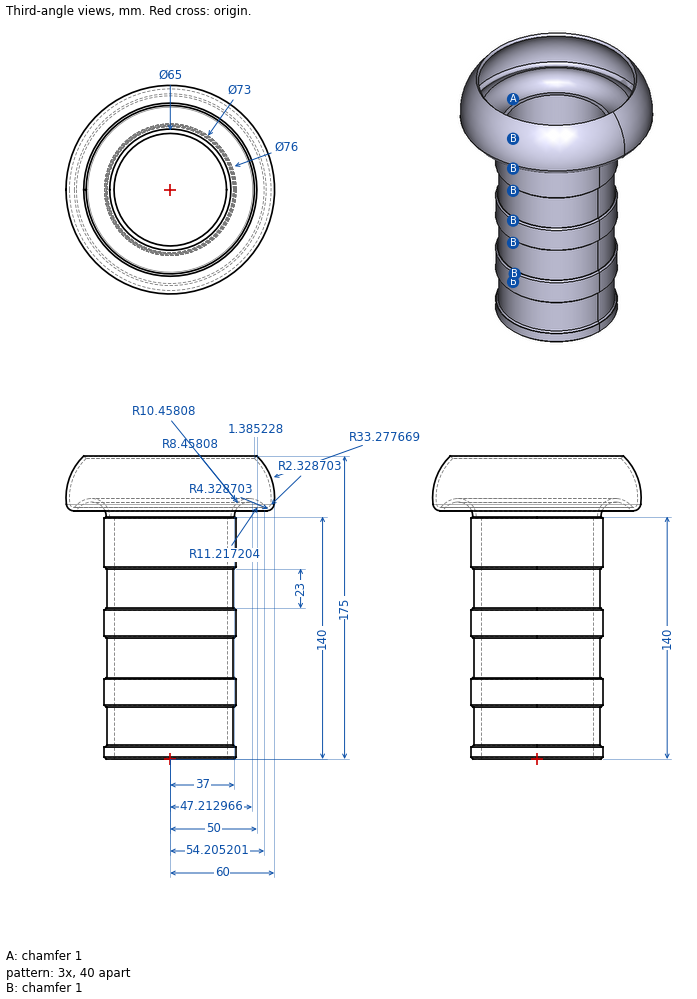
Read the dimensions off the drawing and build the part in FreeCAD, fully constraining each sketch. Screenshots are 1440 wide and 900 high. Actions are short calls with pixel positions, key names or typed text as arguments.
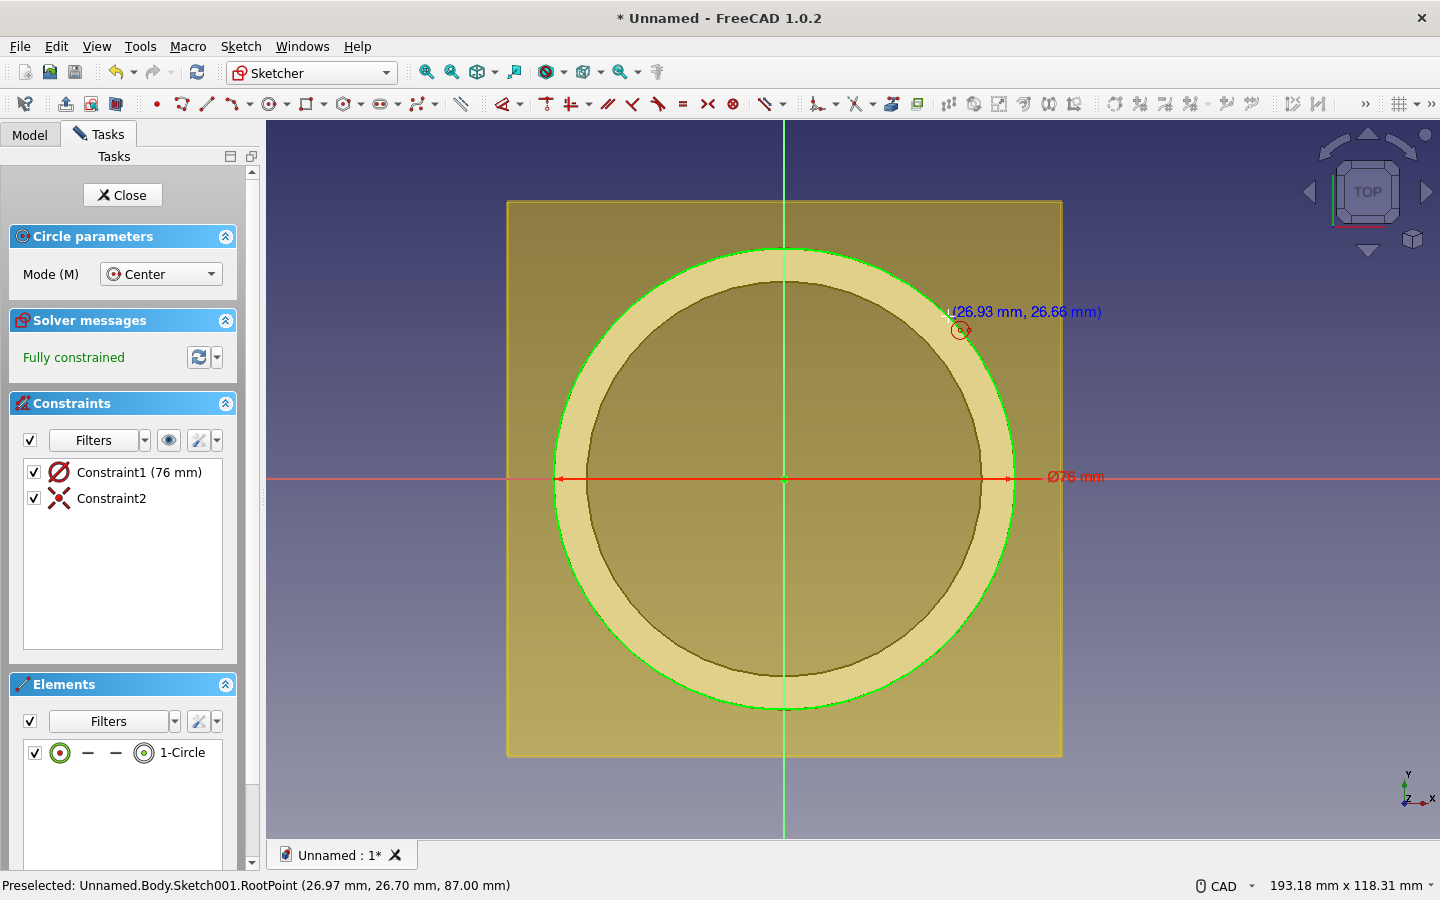
click(784, 479)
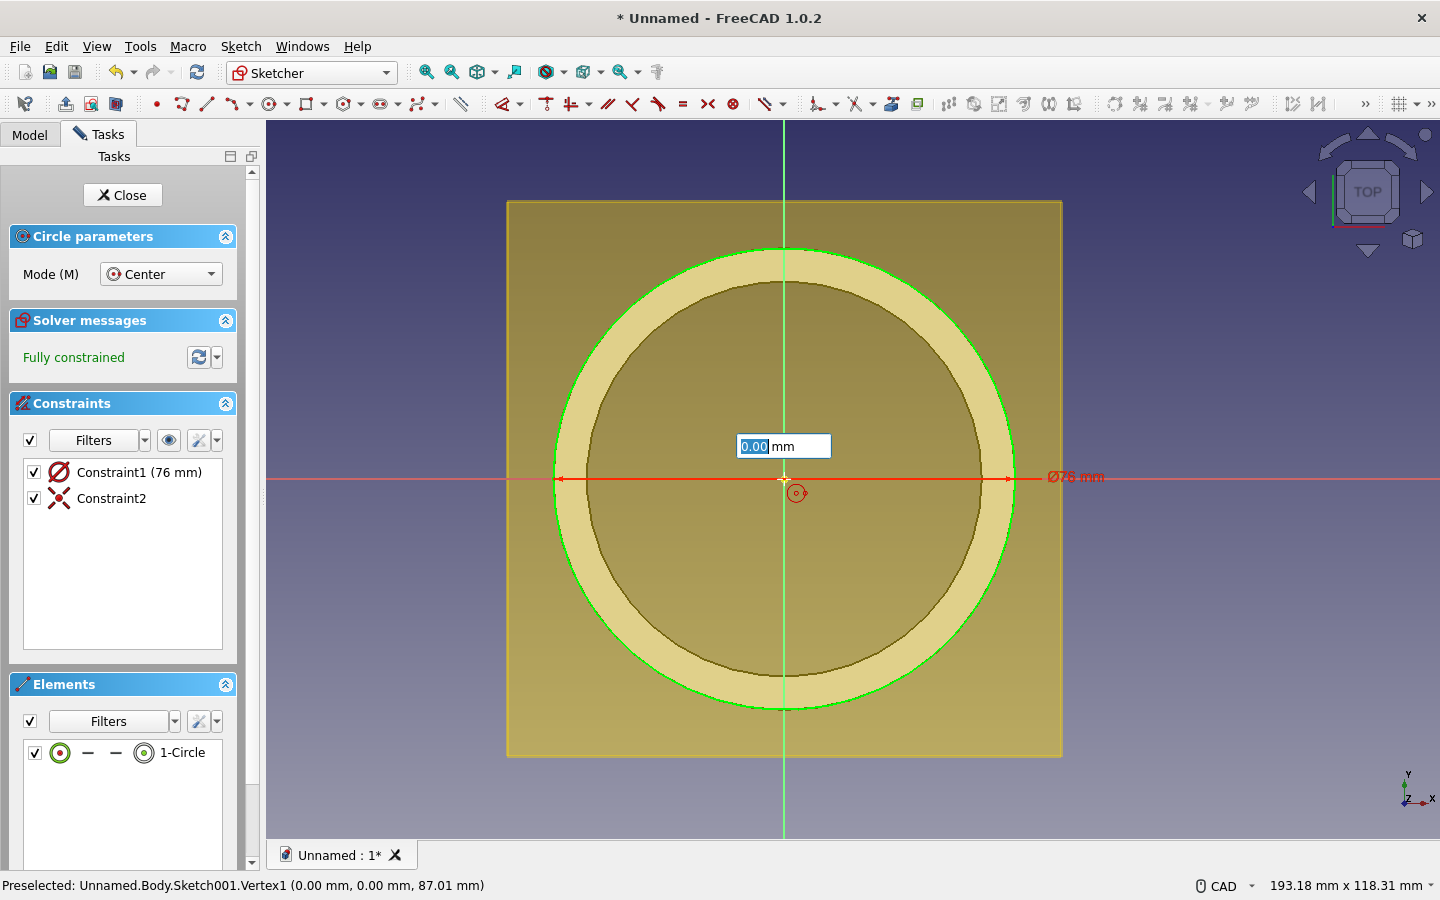
scroll(860, 271, up, 3)
move(860, 270)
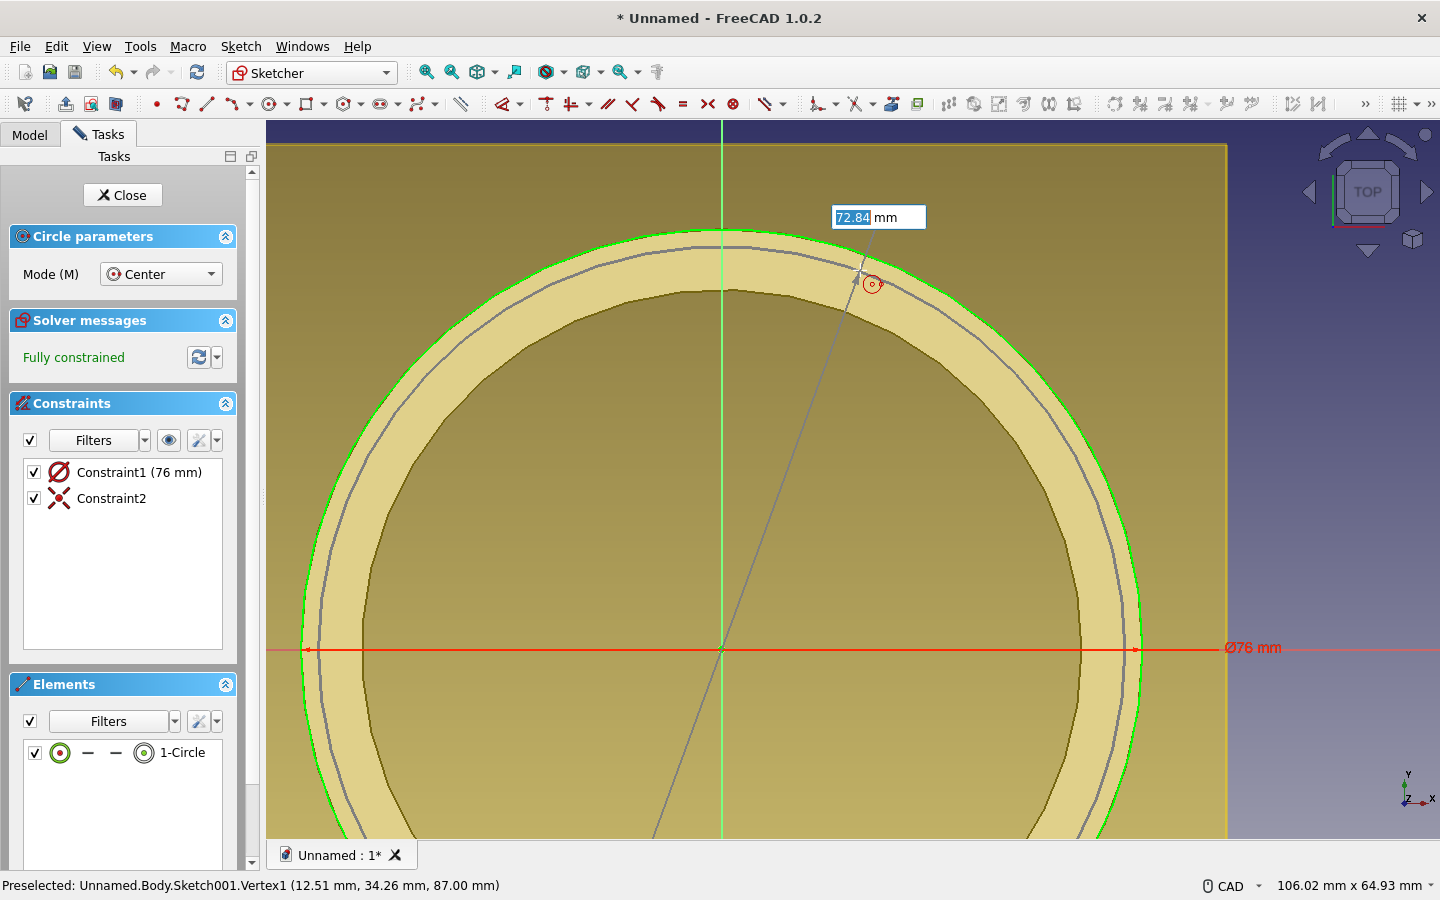
text(73)
key(Return)
key(Escape)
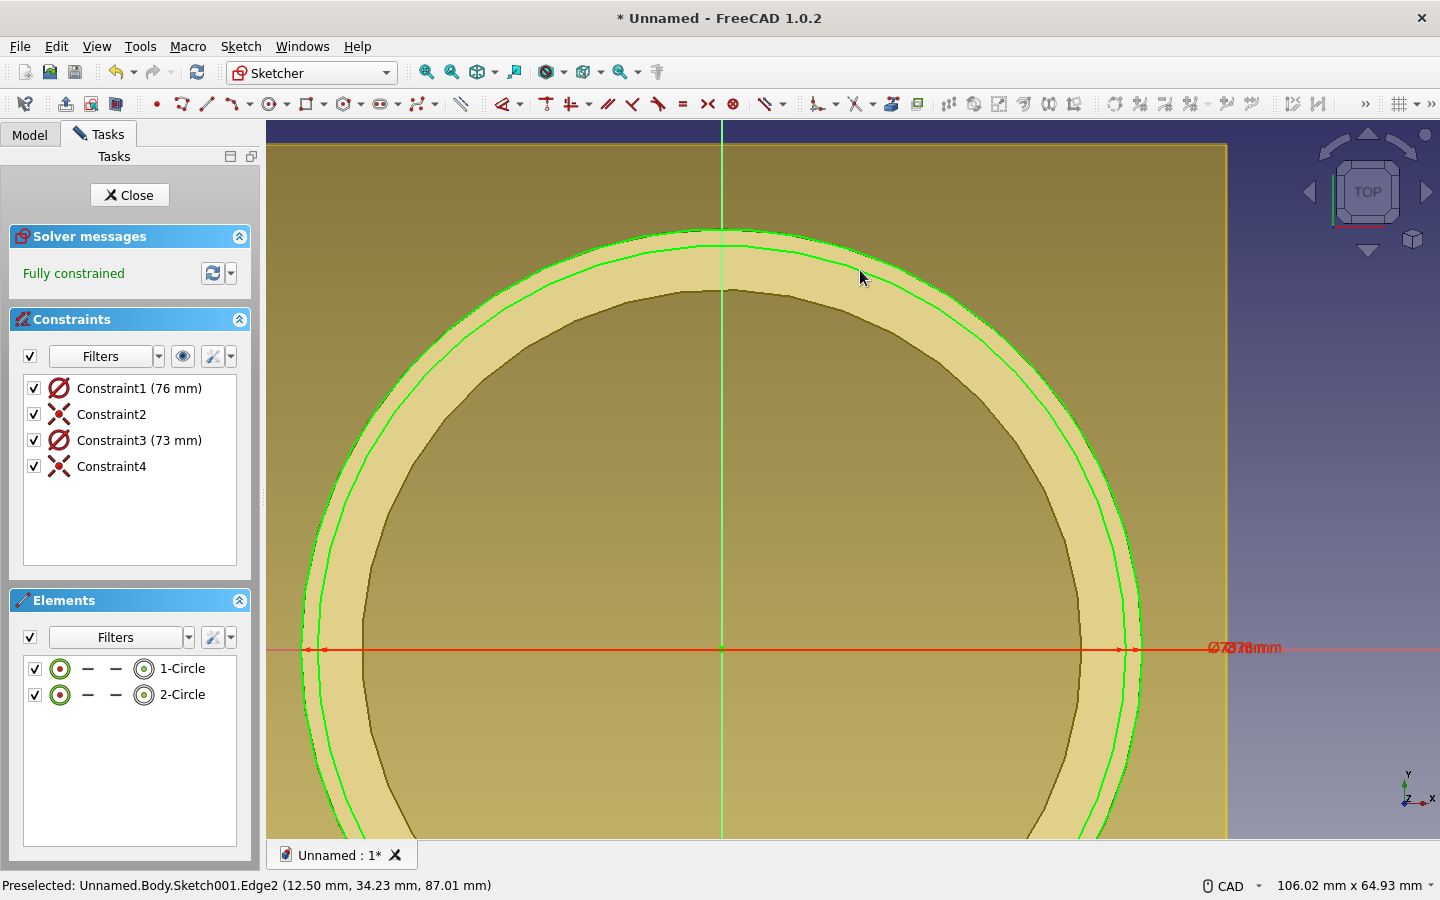
click(130, 195)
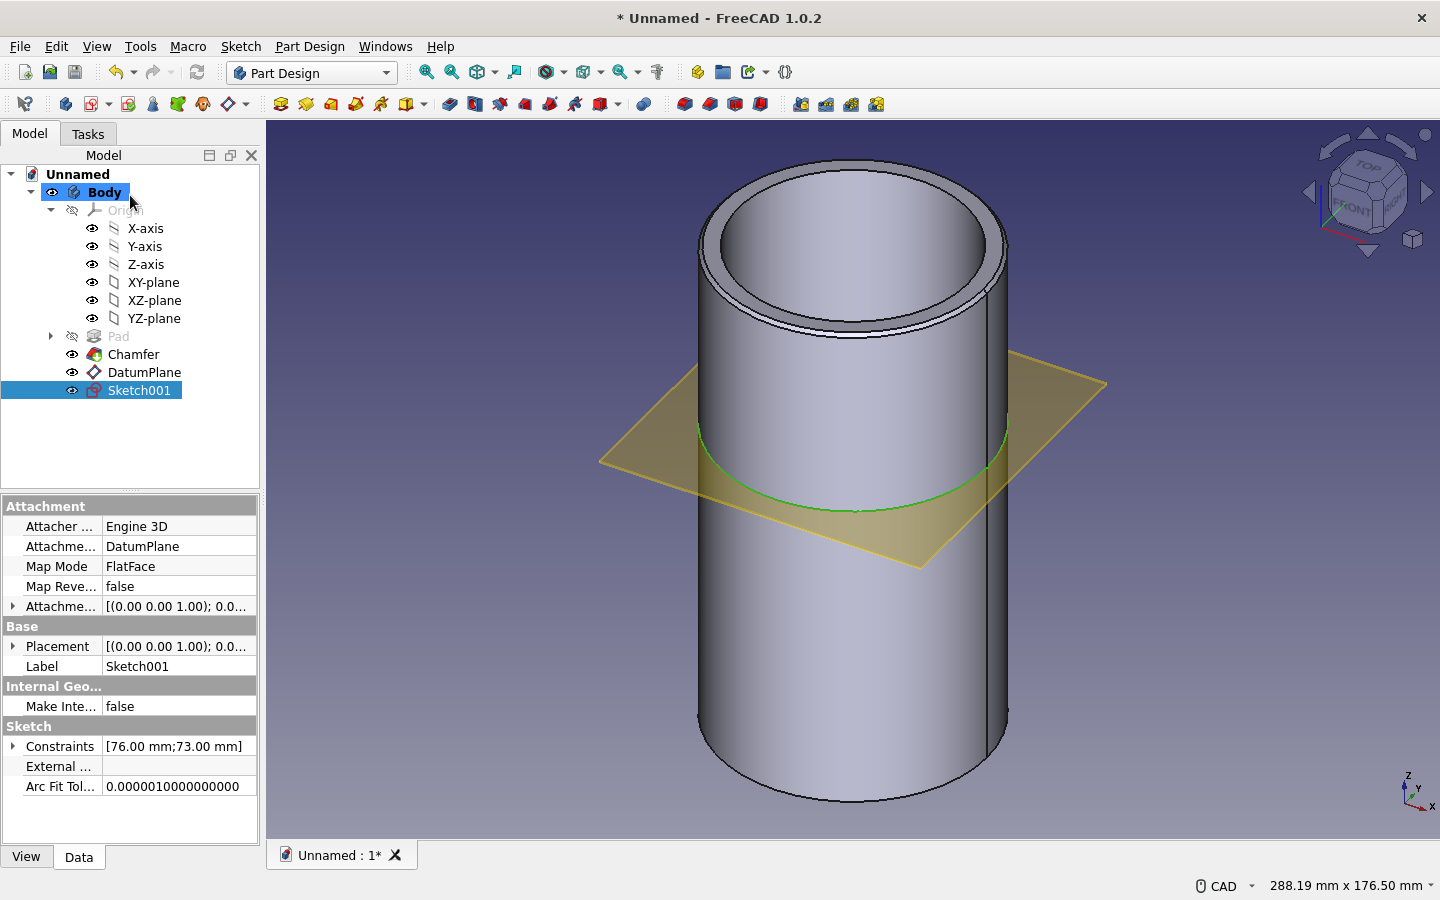
click(450, 104)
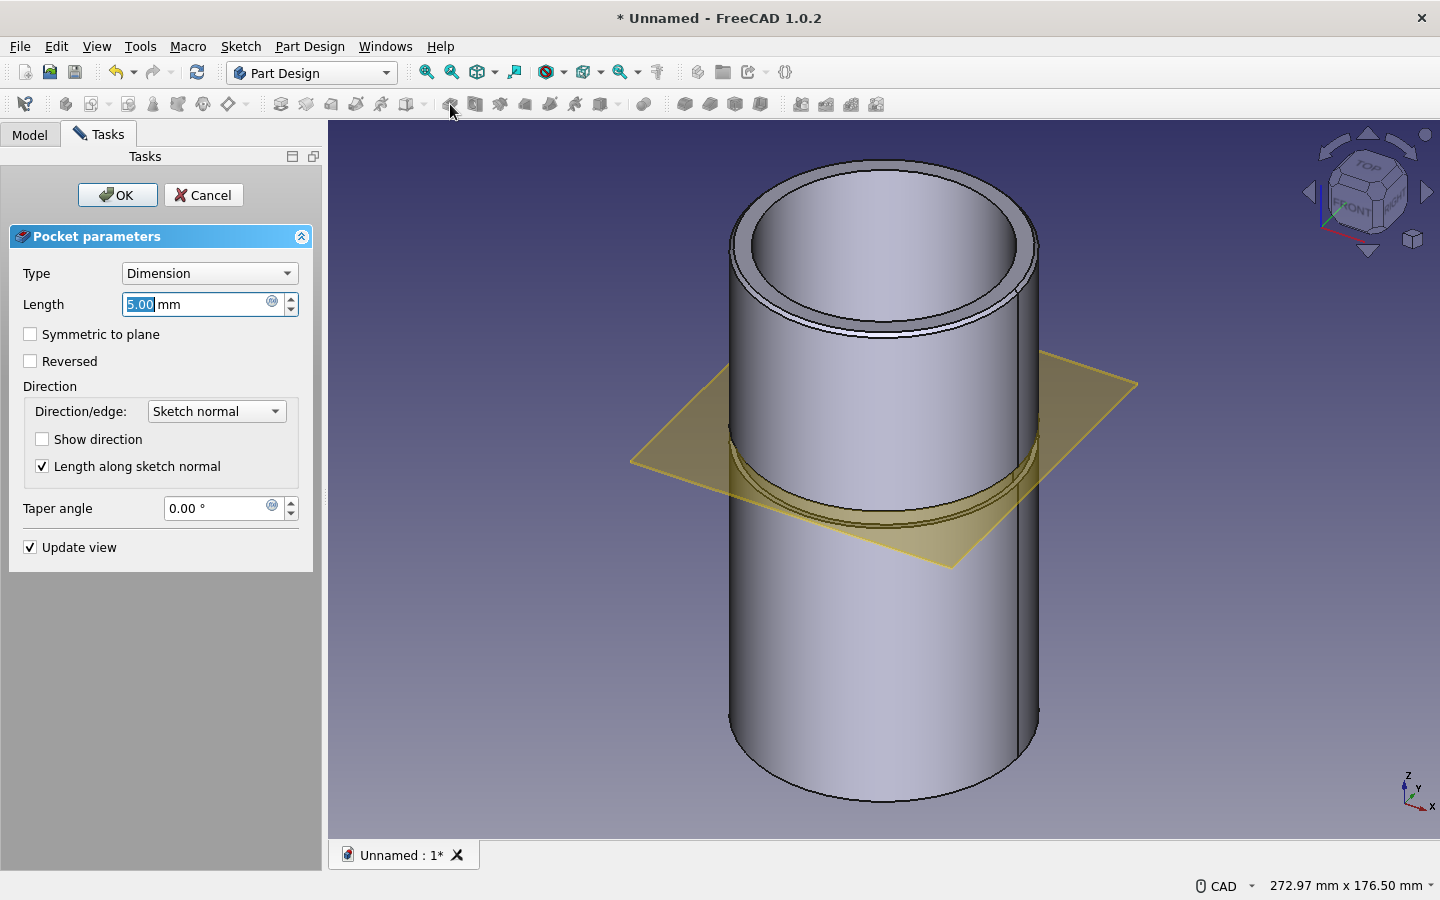
text(23)
key(Tab)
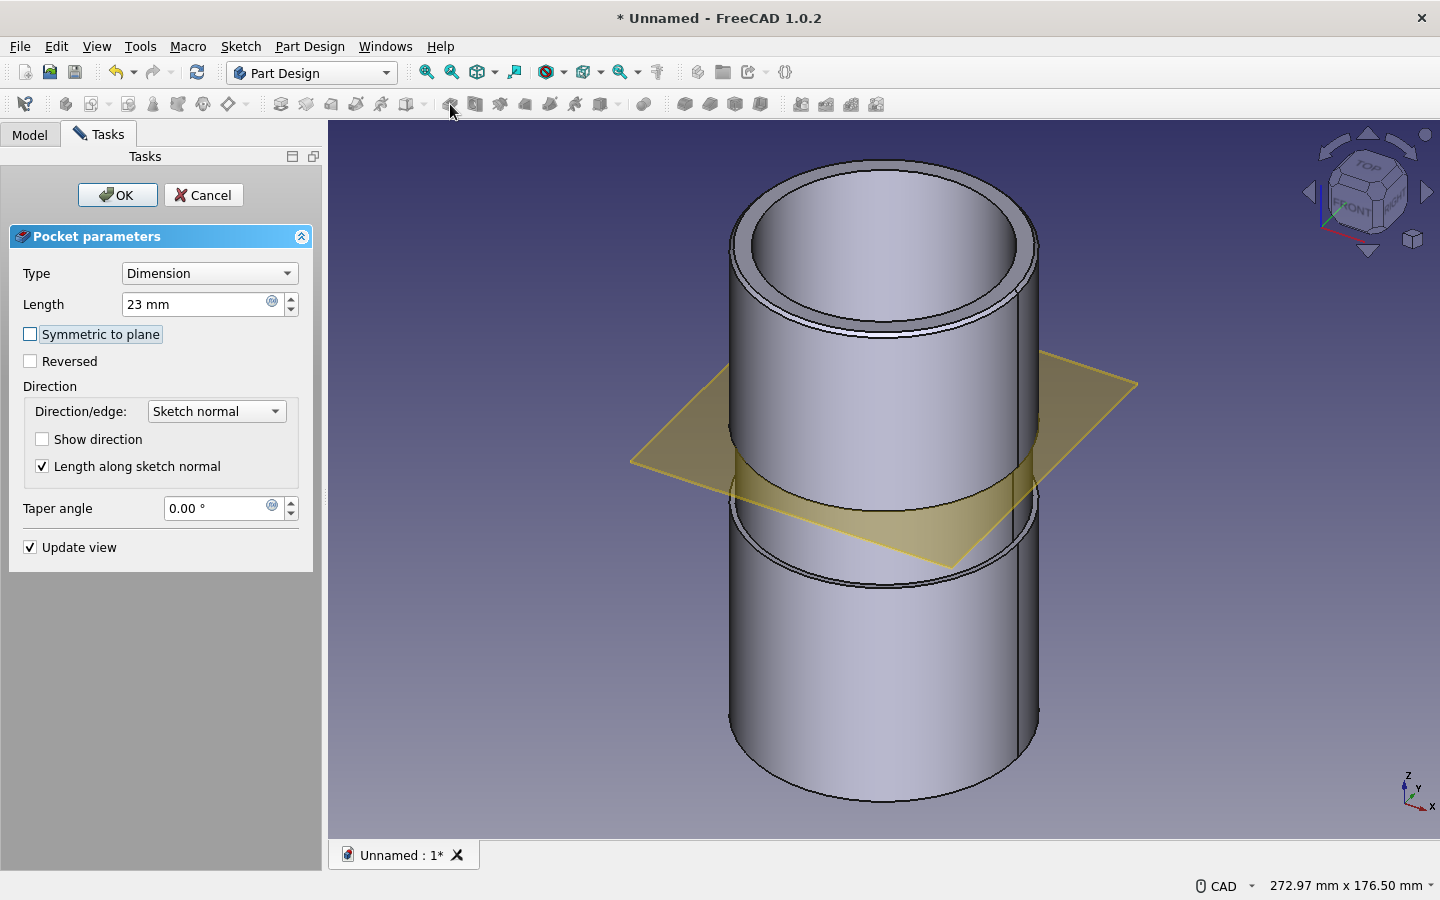
click(31, 361)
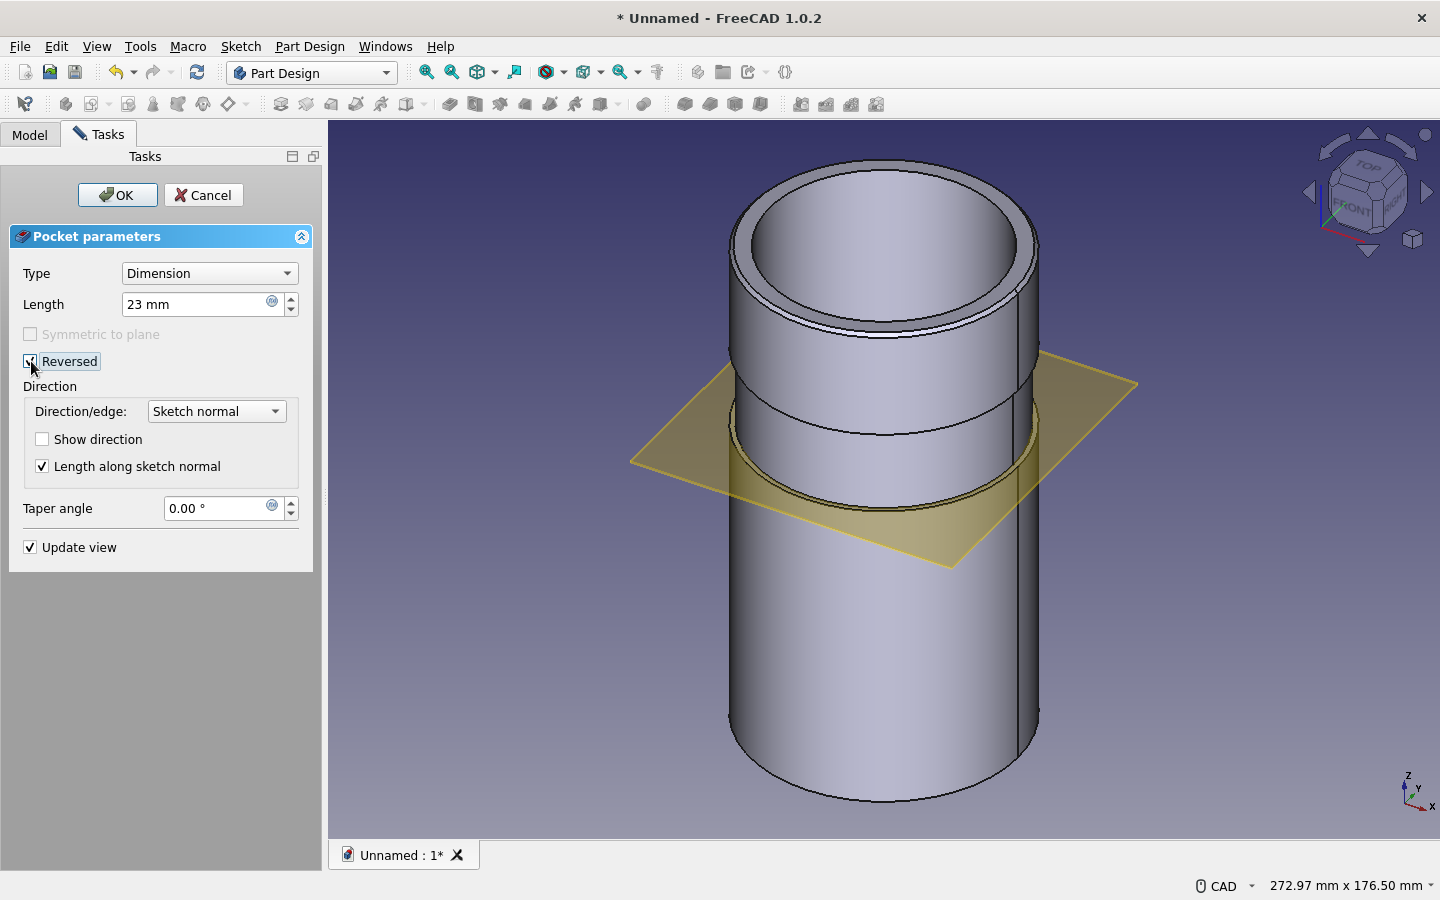
click(118, 195)